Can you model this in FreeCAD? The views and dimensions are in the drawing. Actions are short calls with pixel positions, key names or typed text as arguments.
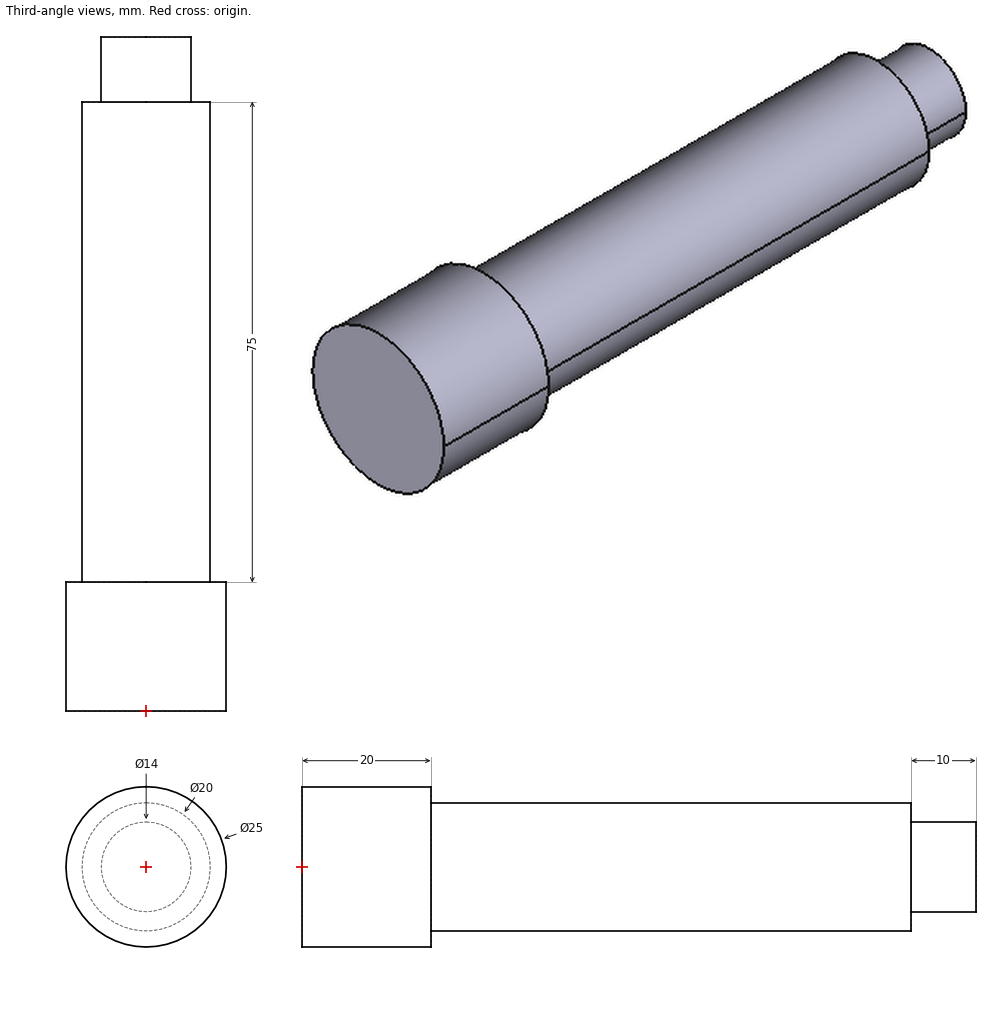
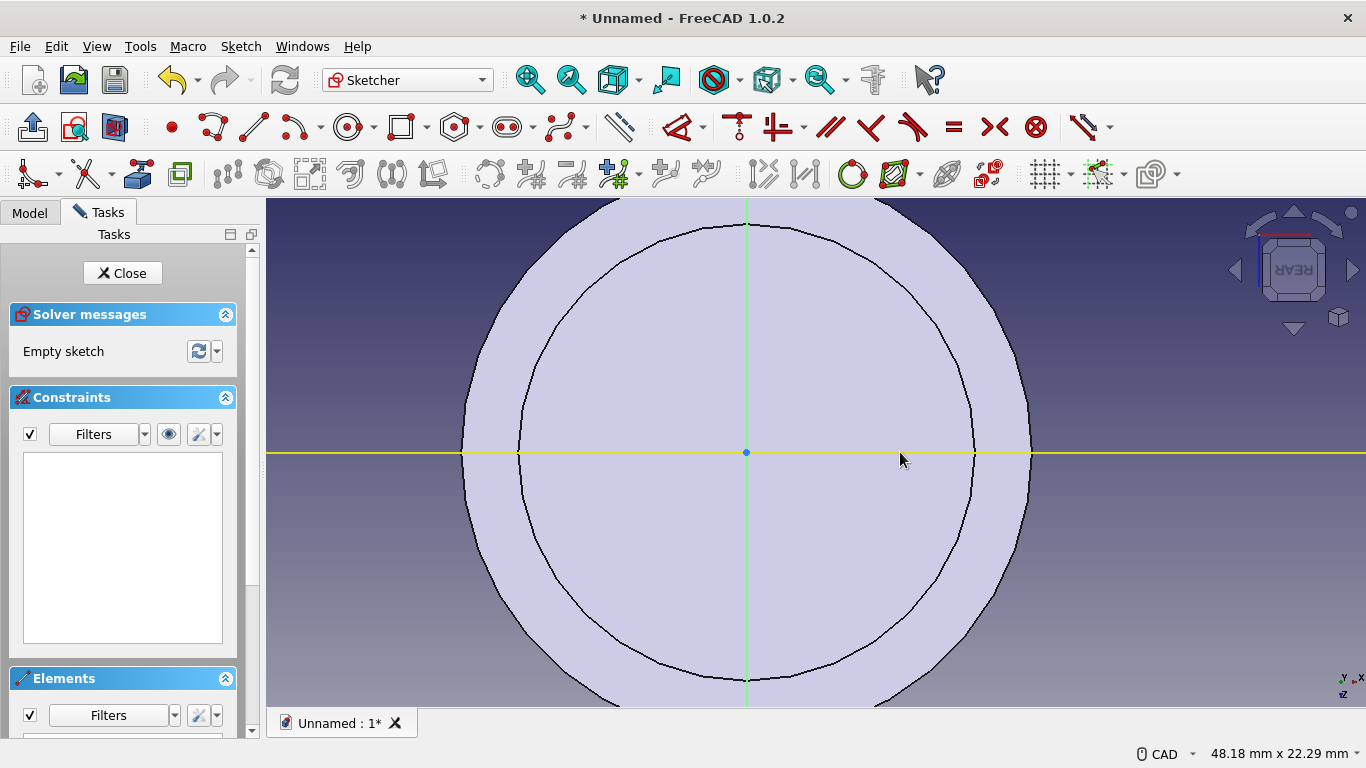
click(348, 128)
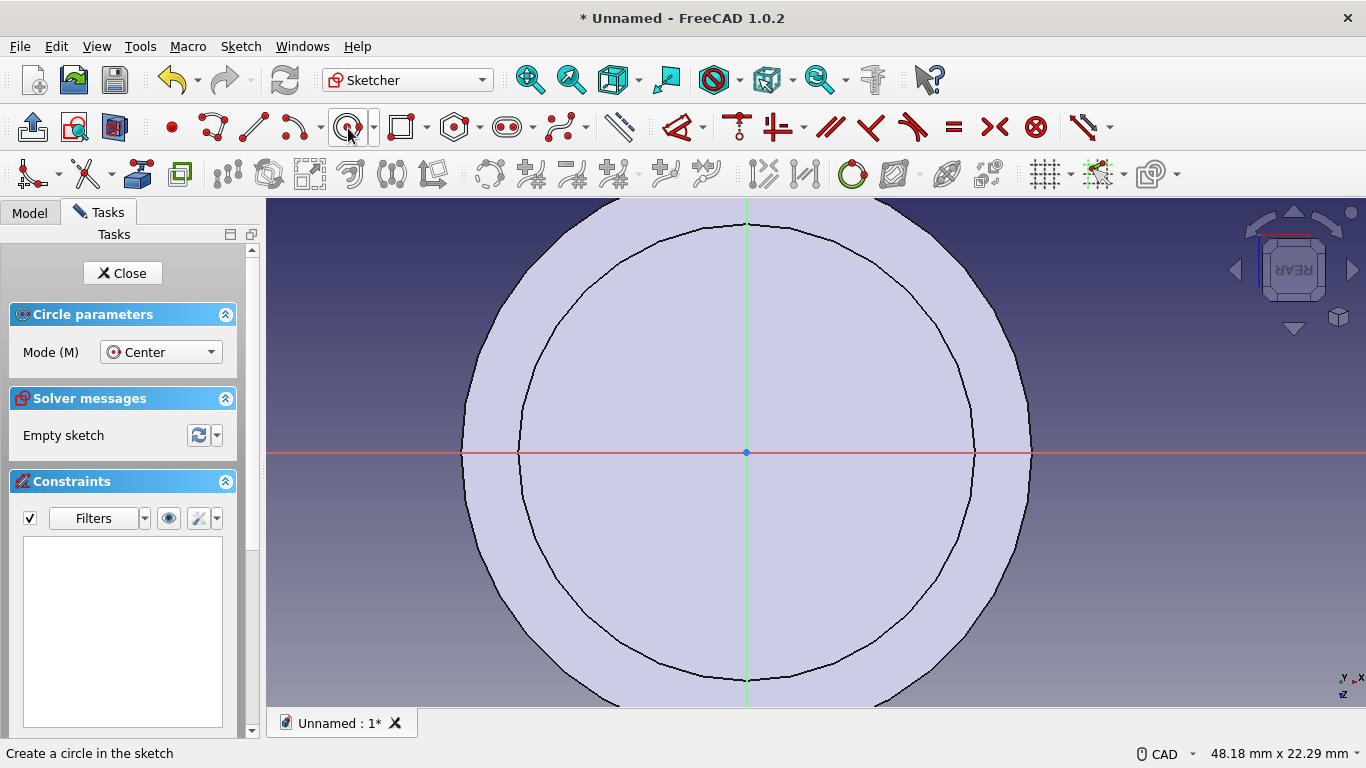
click(747, 452)
move(860, 339)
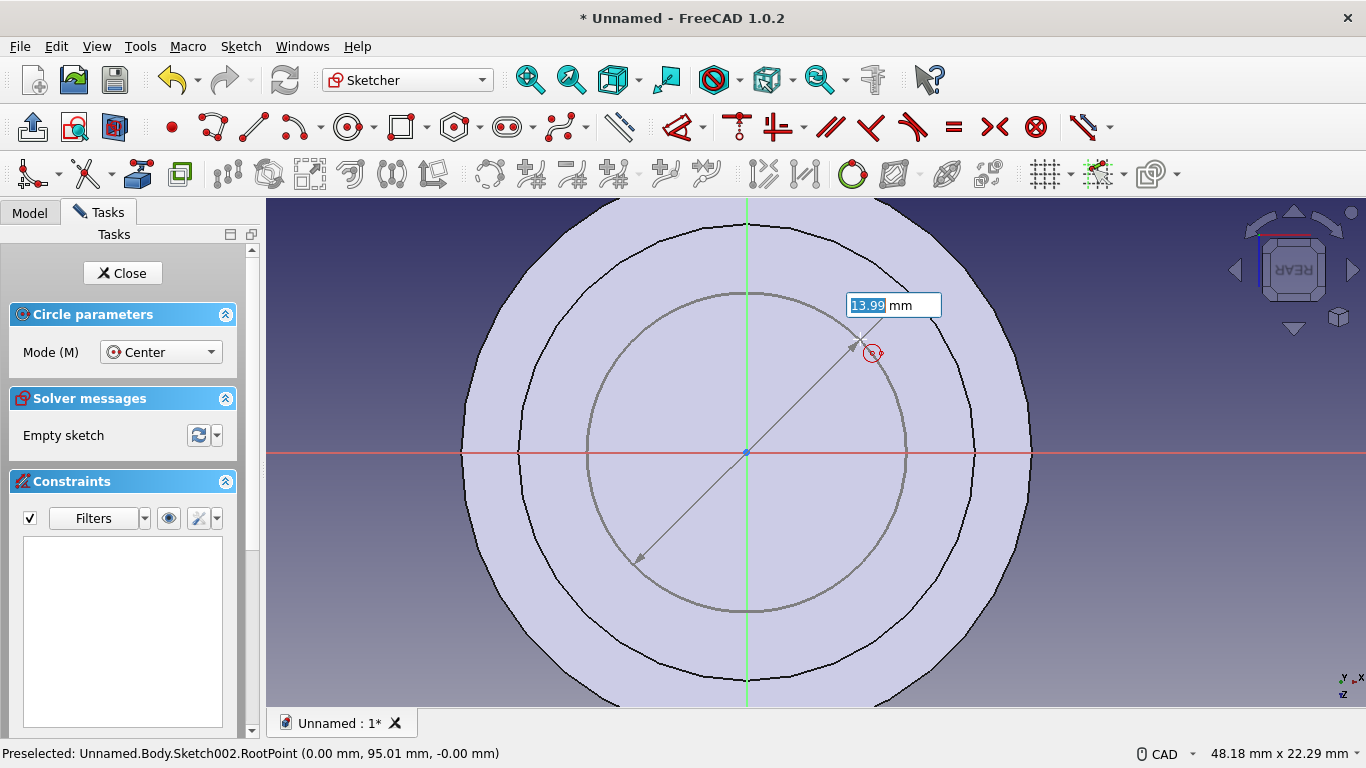
text(14)
key(Return)
key(Escape)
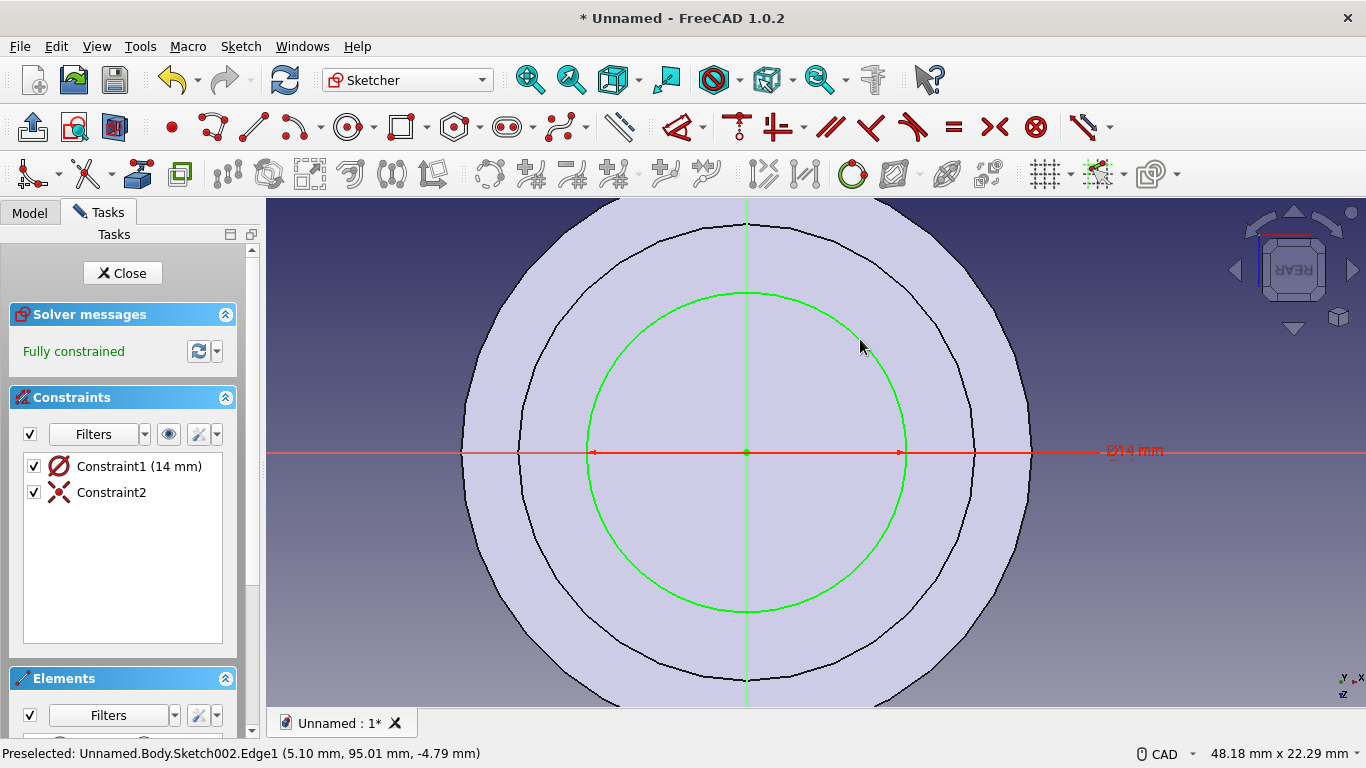
click(123, 273)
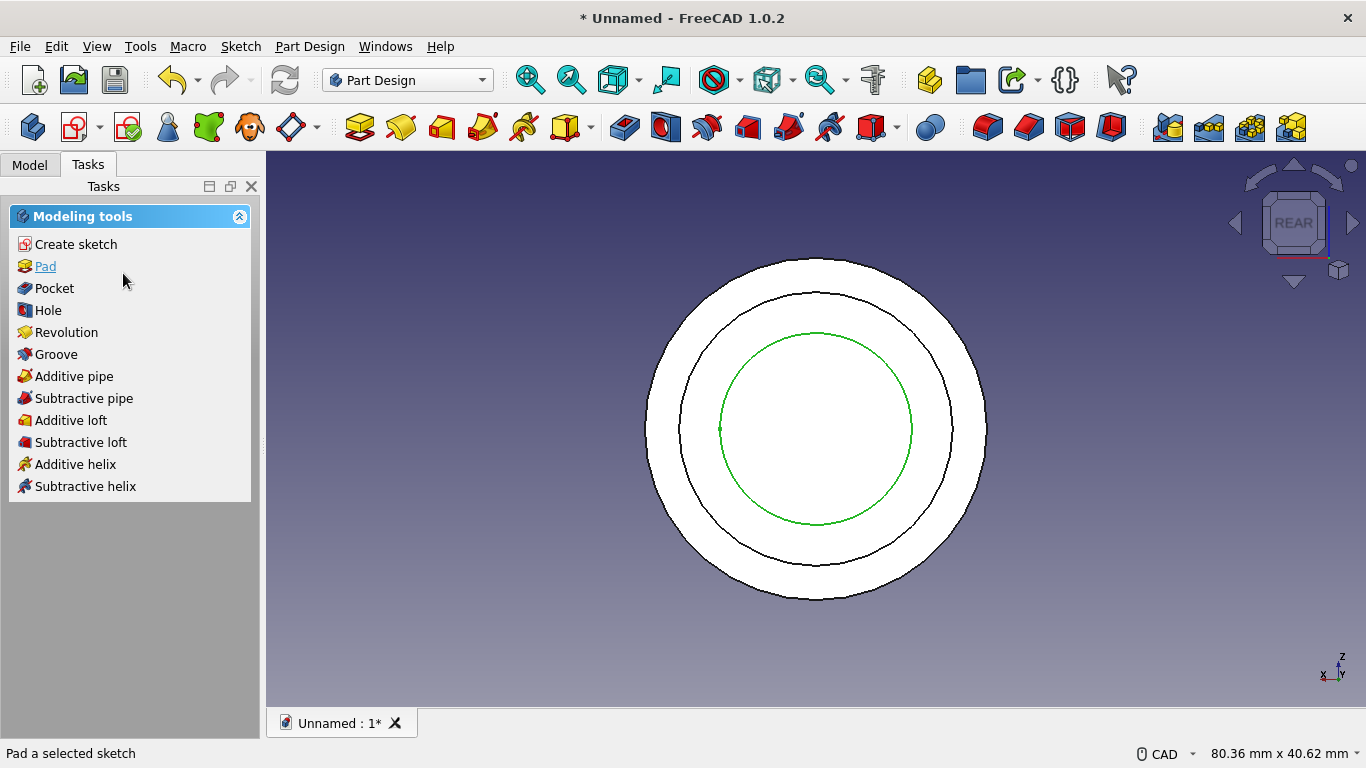
click(360, 128)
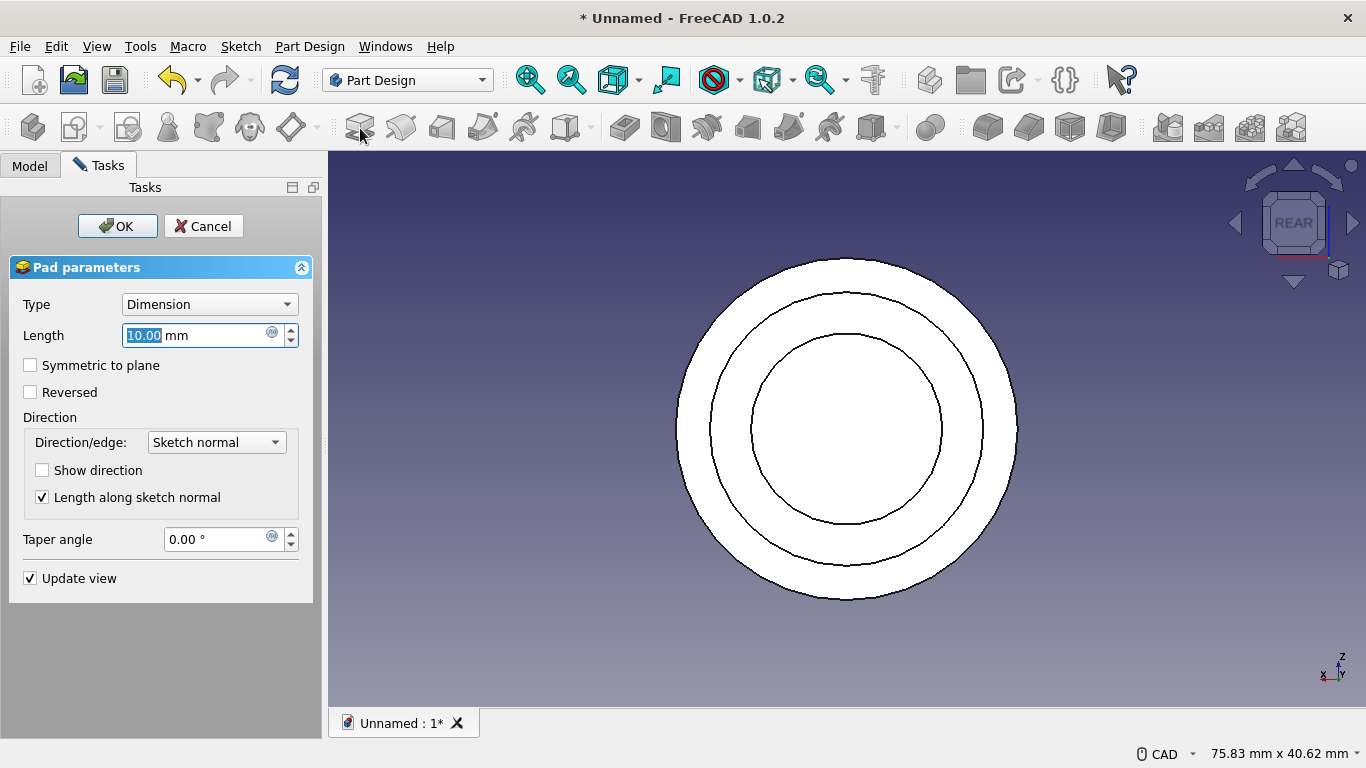
text(10)
key(Tab)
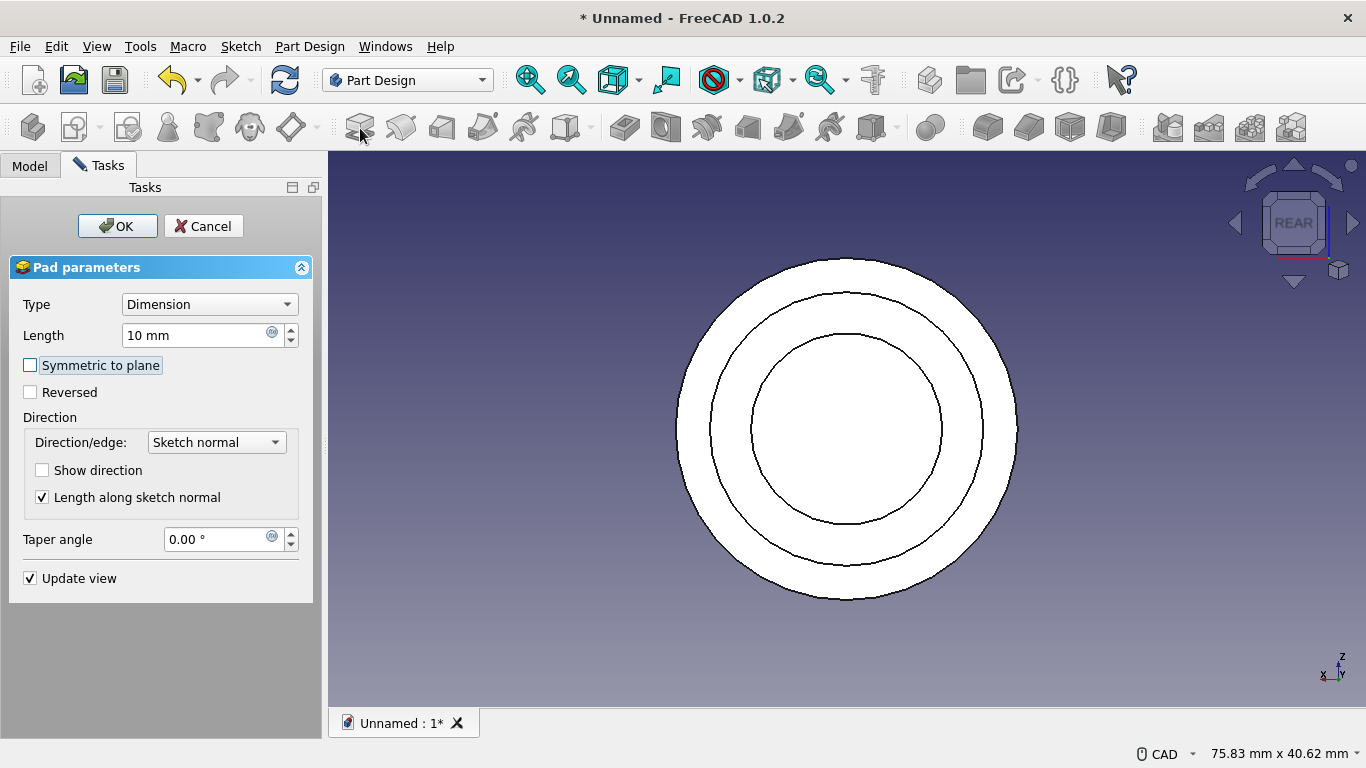
click(118, 226)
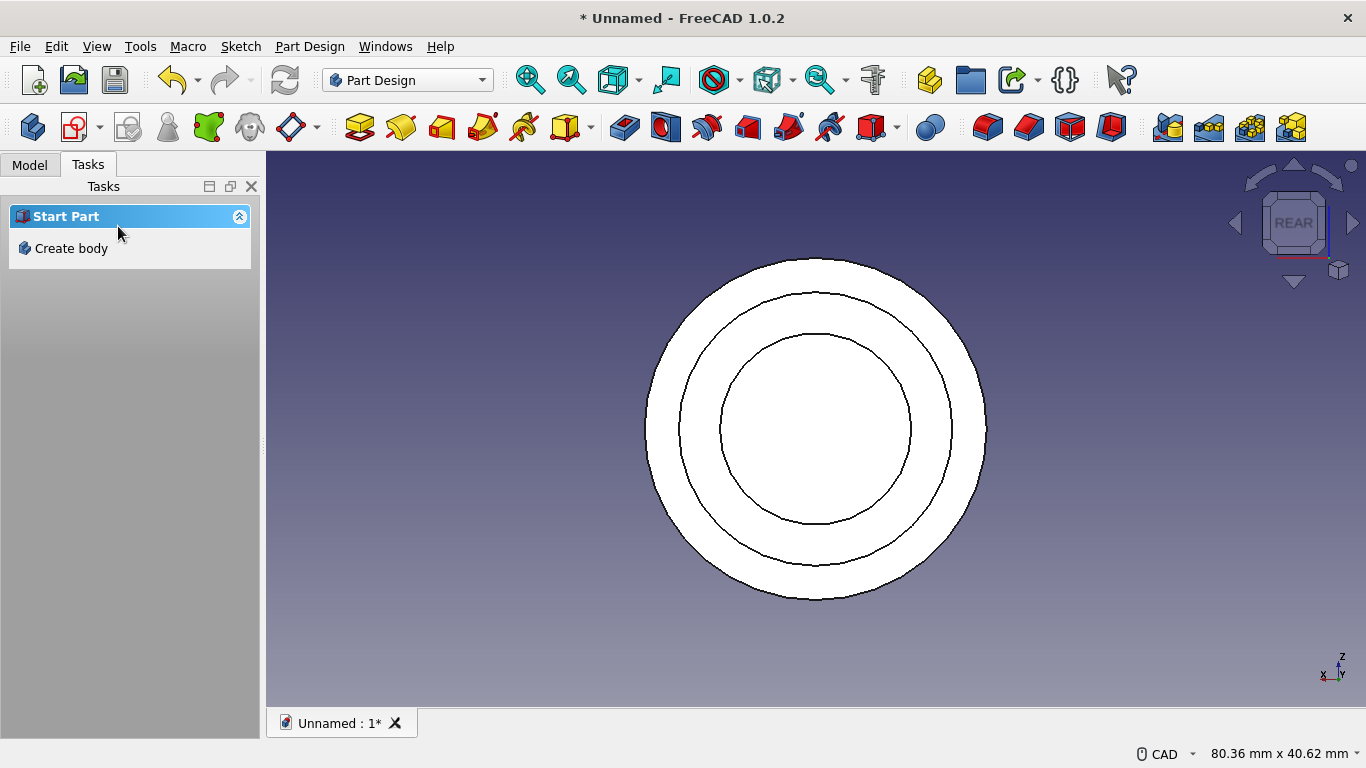
key(0)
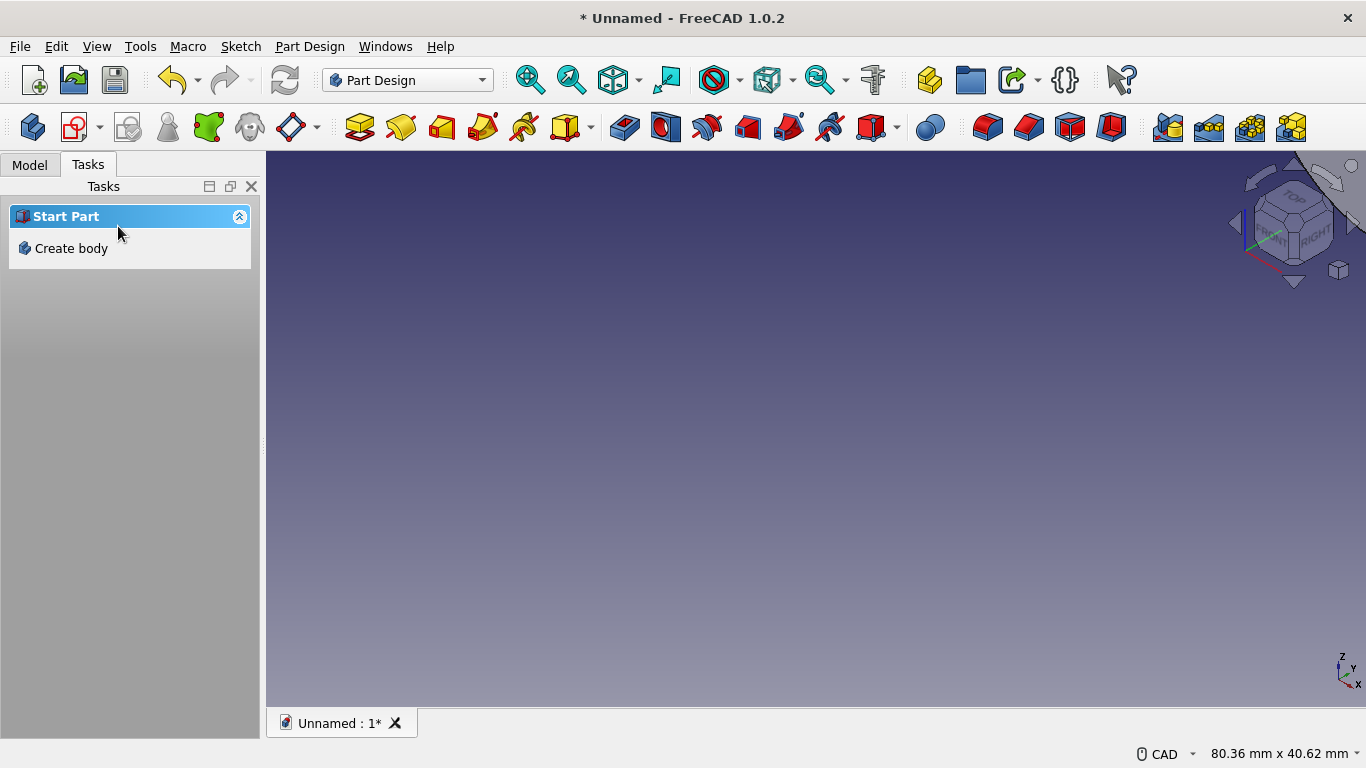
click(531, 80)